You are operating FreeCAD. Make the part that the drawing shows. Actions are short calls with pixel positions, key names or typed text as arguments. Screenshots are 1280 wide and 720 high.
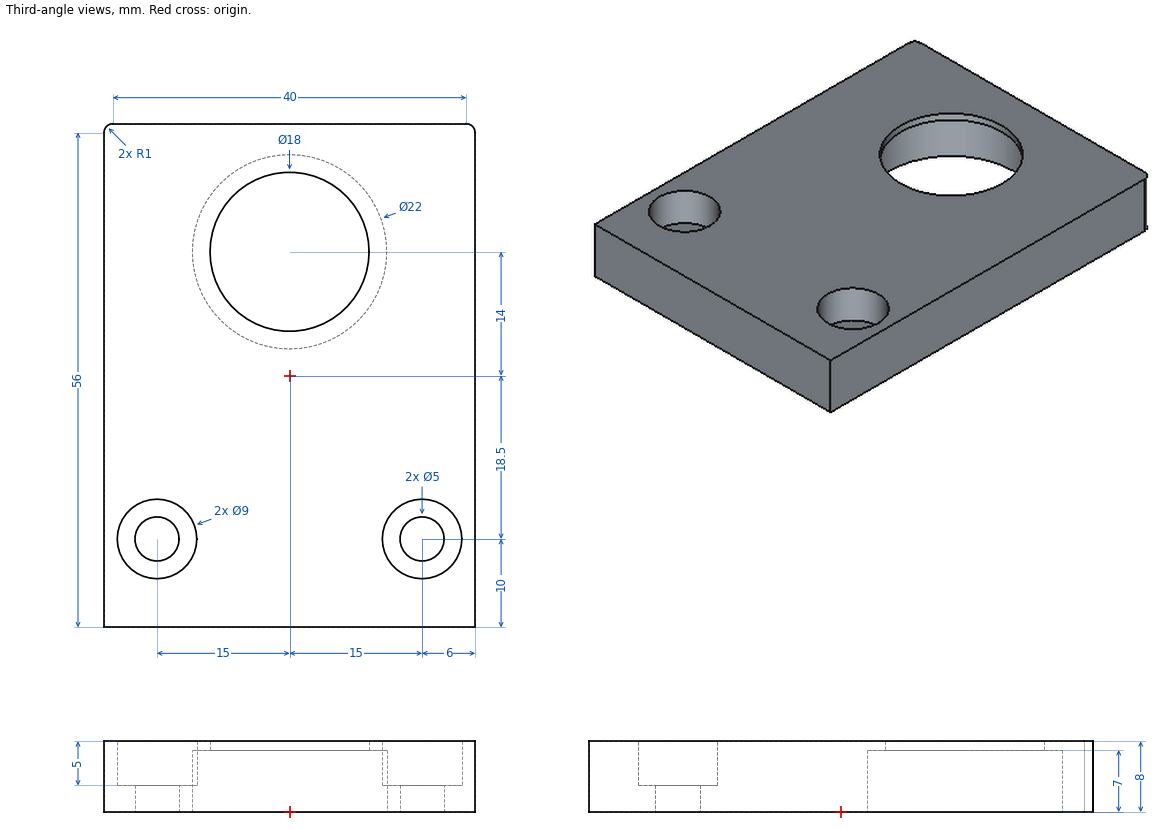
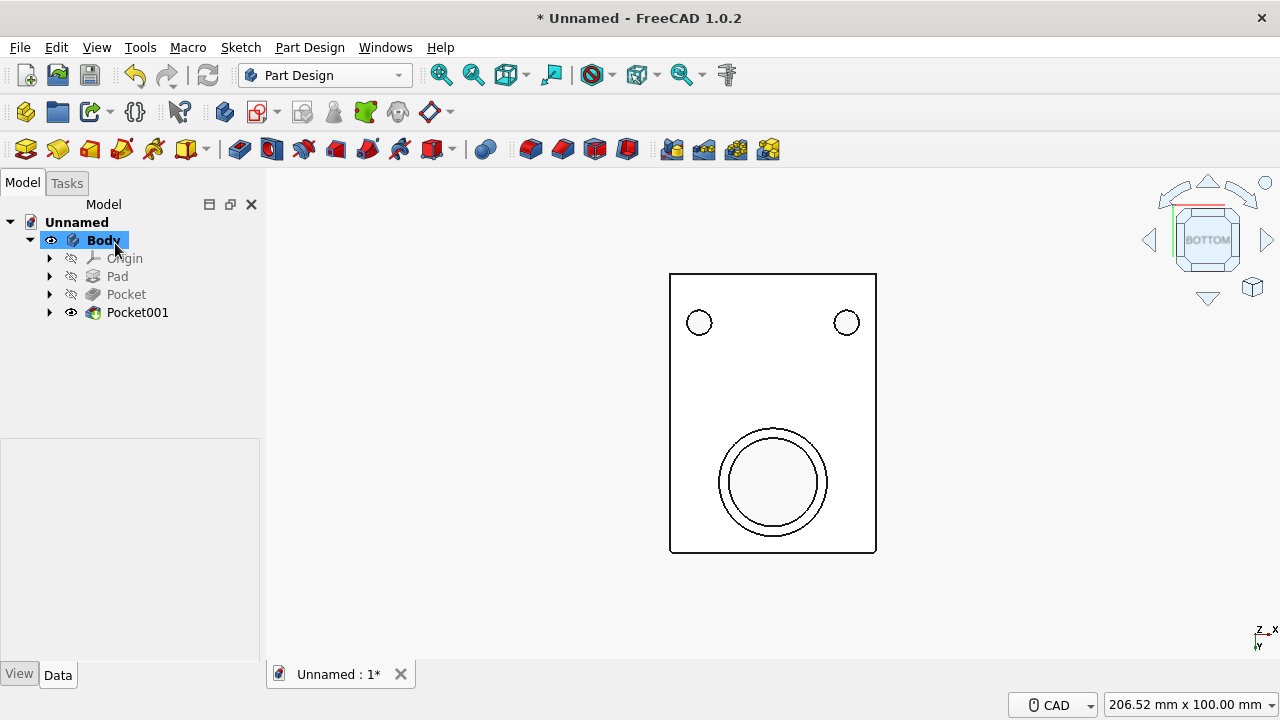
key(0)